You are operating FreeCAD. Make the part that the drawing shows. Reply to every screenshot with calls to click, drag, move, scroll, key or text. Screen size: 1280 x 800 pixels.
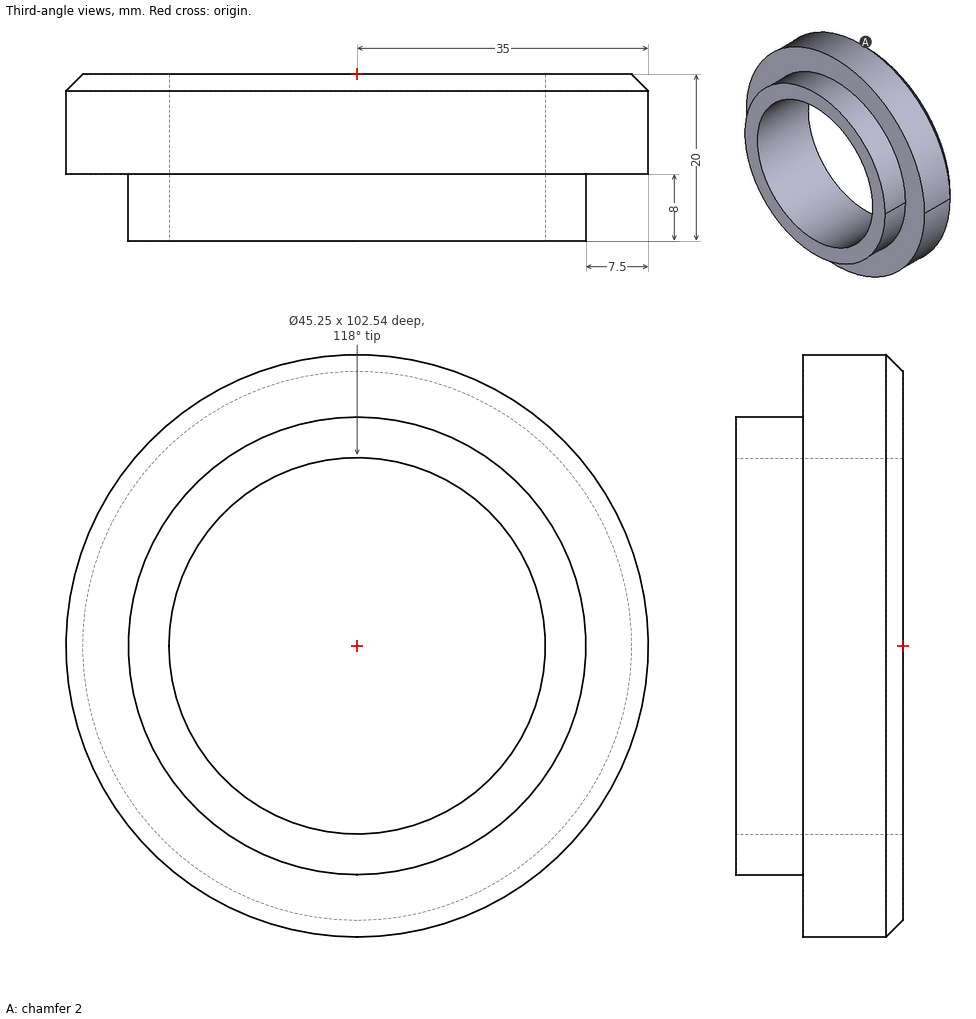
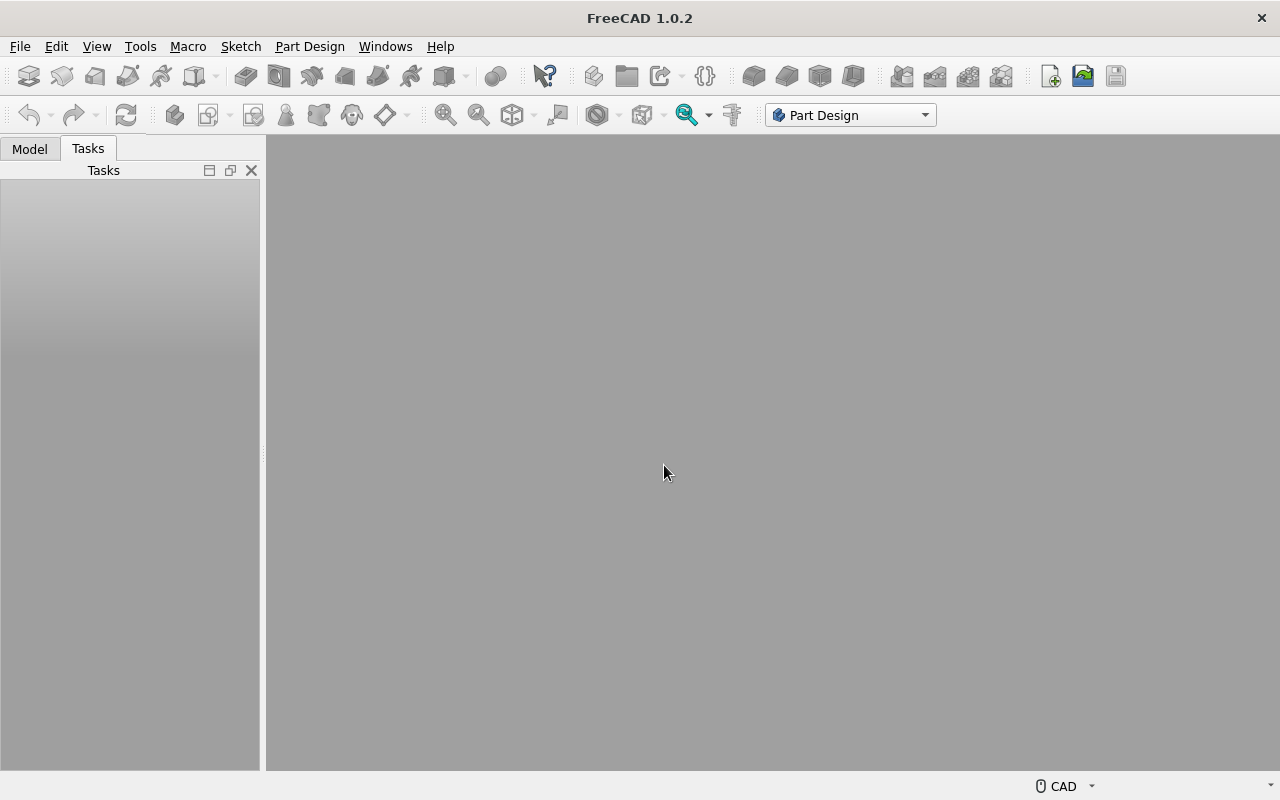
click(1050, 76)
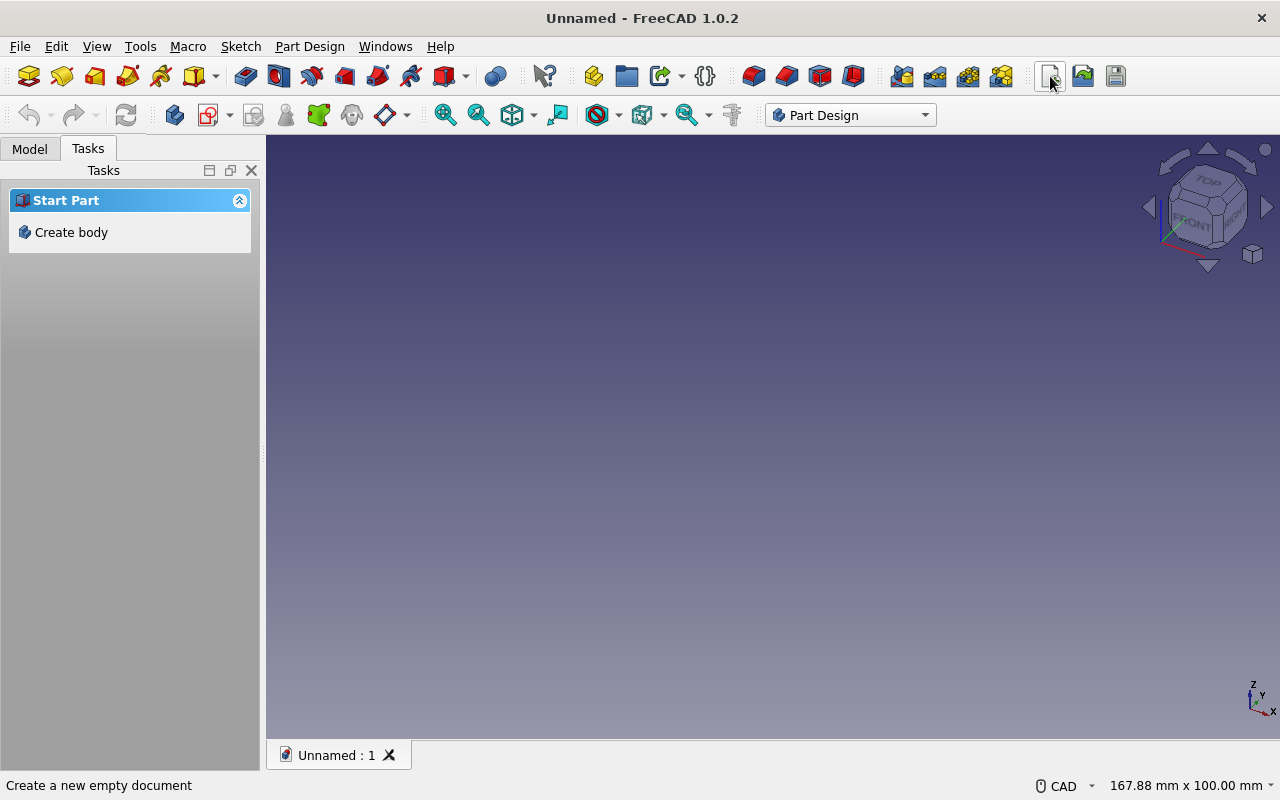
click(208, 116)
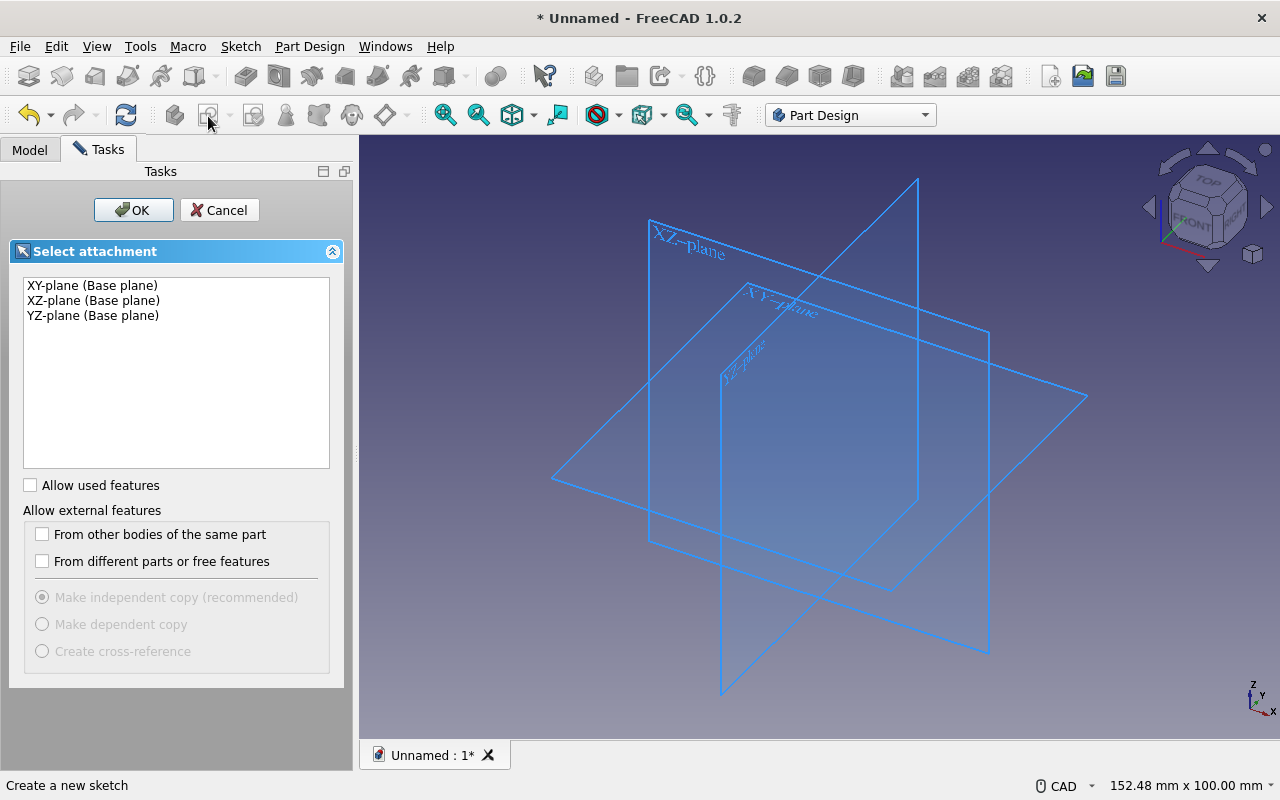
click(84, 286)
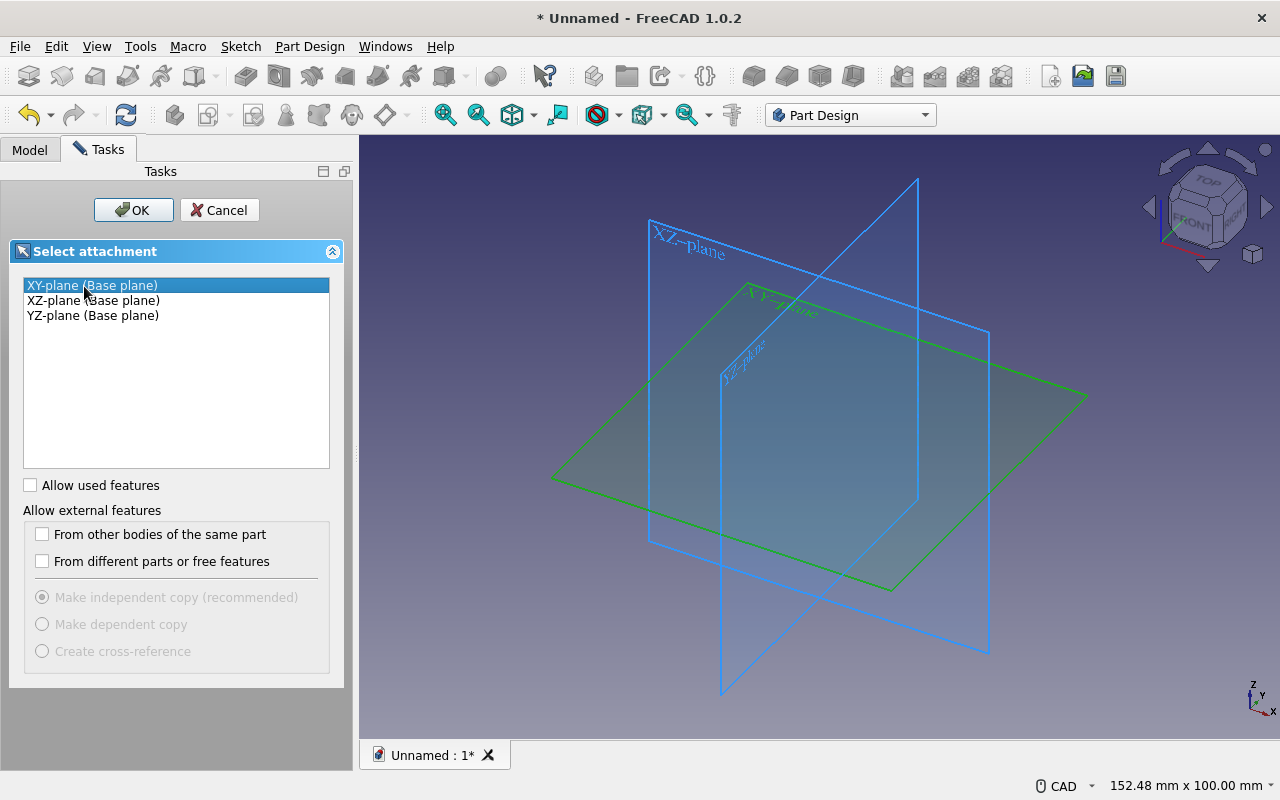
click(134, 210)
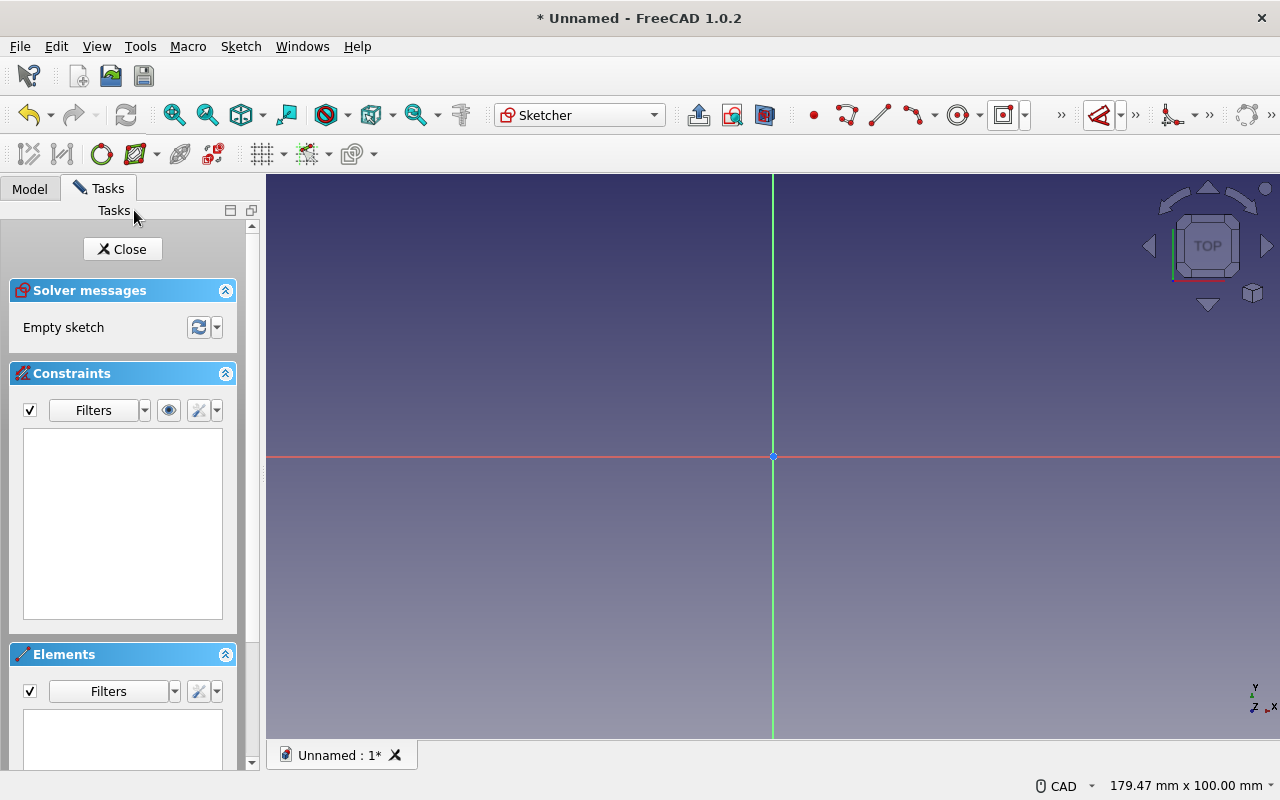
scroll(969, 546, up, 5)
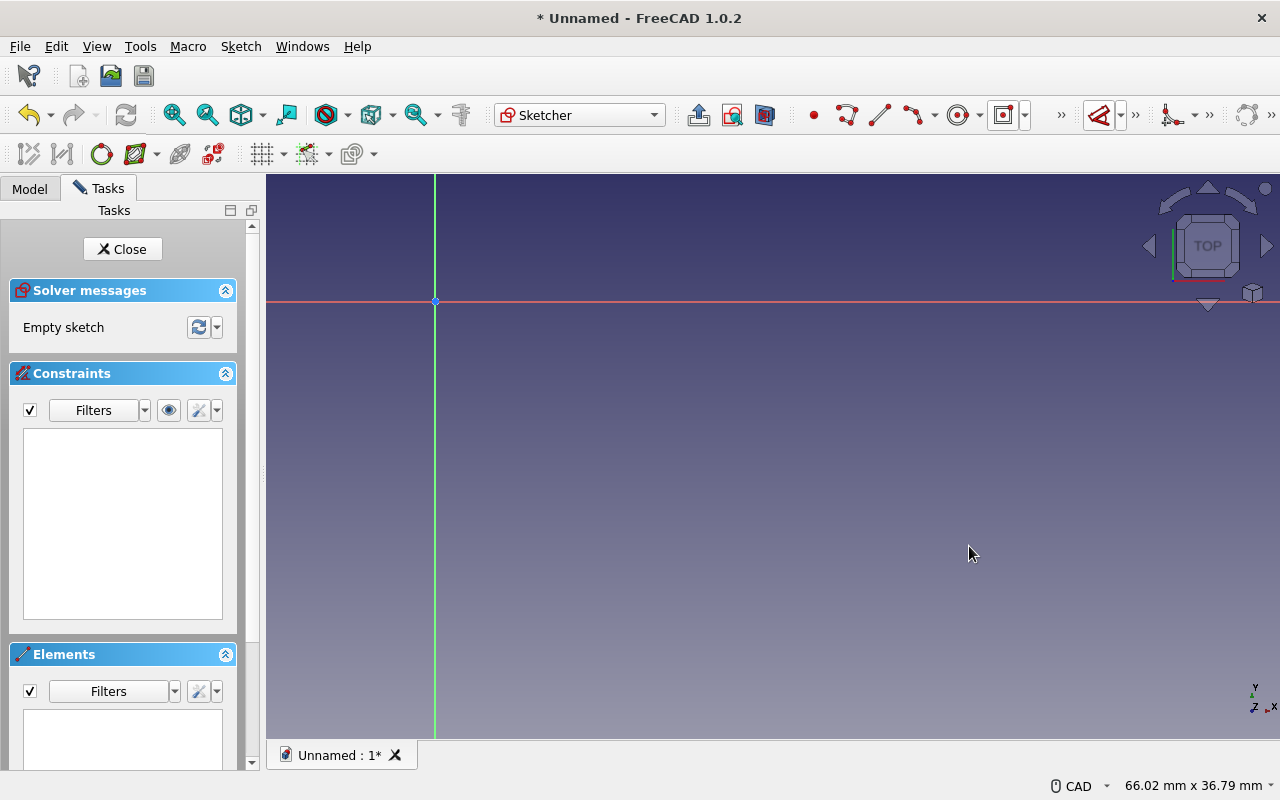
click(847, 116)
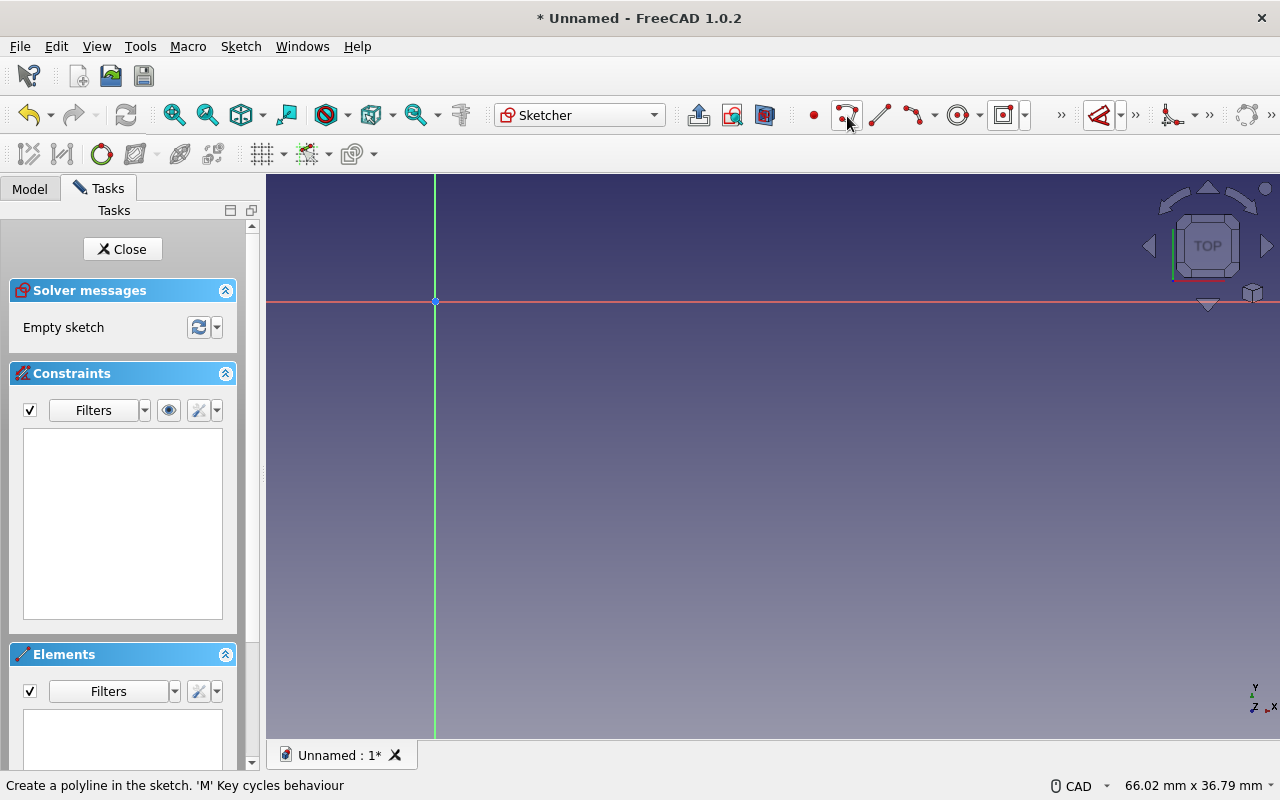
click(435, 302)
click(444, 609)
click(857, 609)
click(857, 486)
click(973, 486)
click(973, 311)
click(435, 302)
key(Escape)
key(Escape)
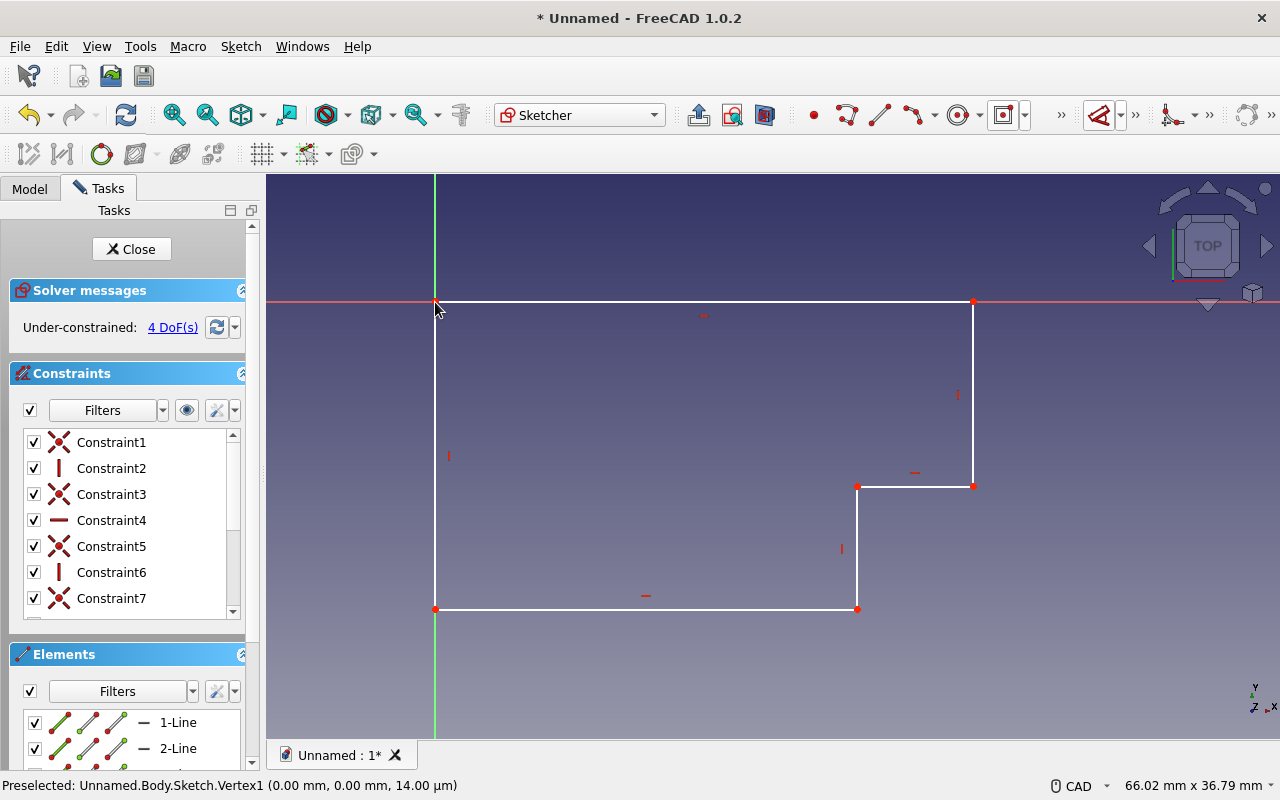
click(857, 573)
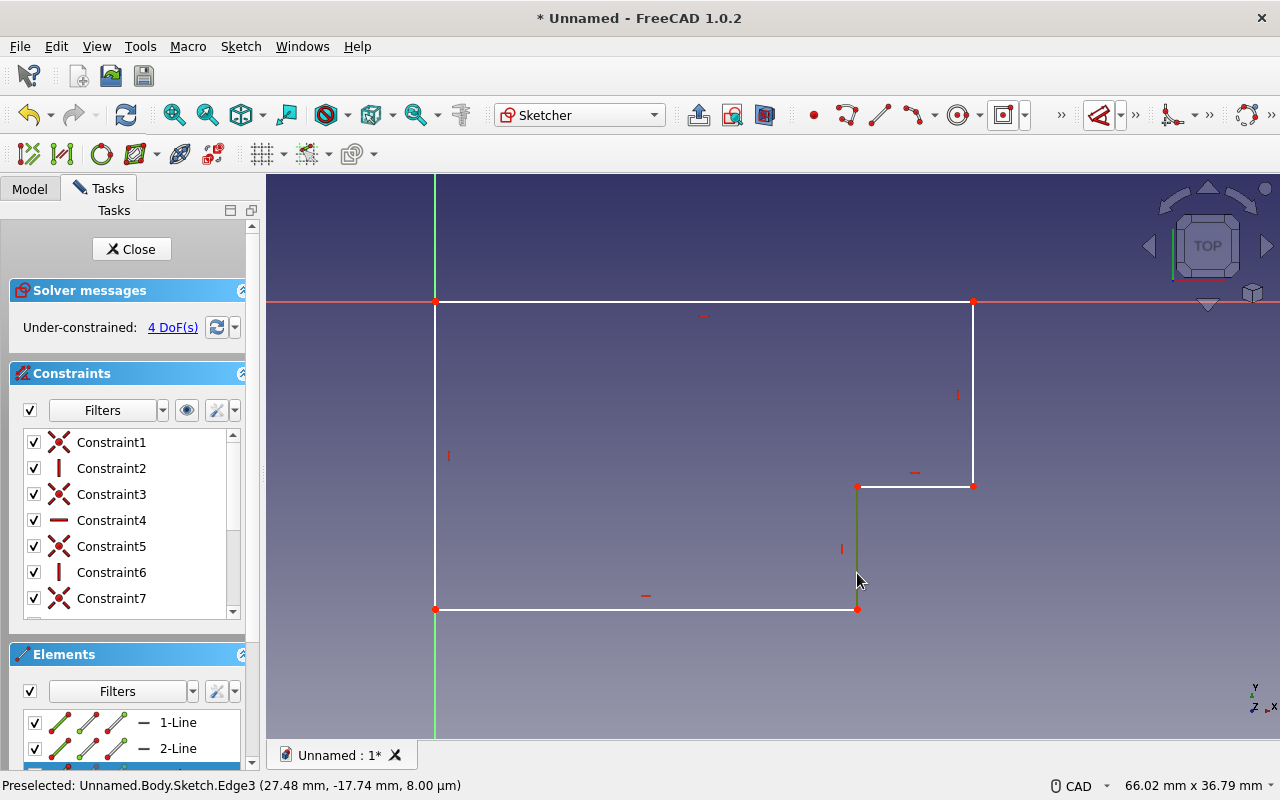
click(1120, 116)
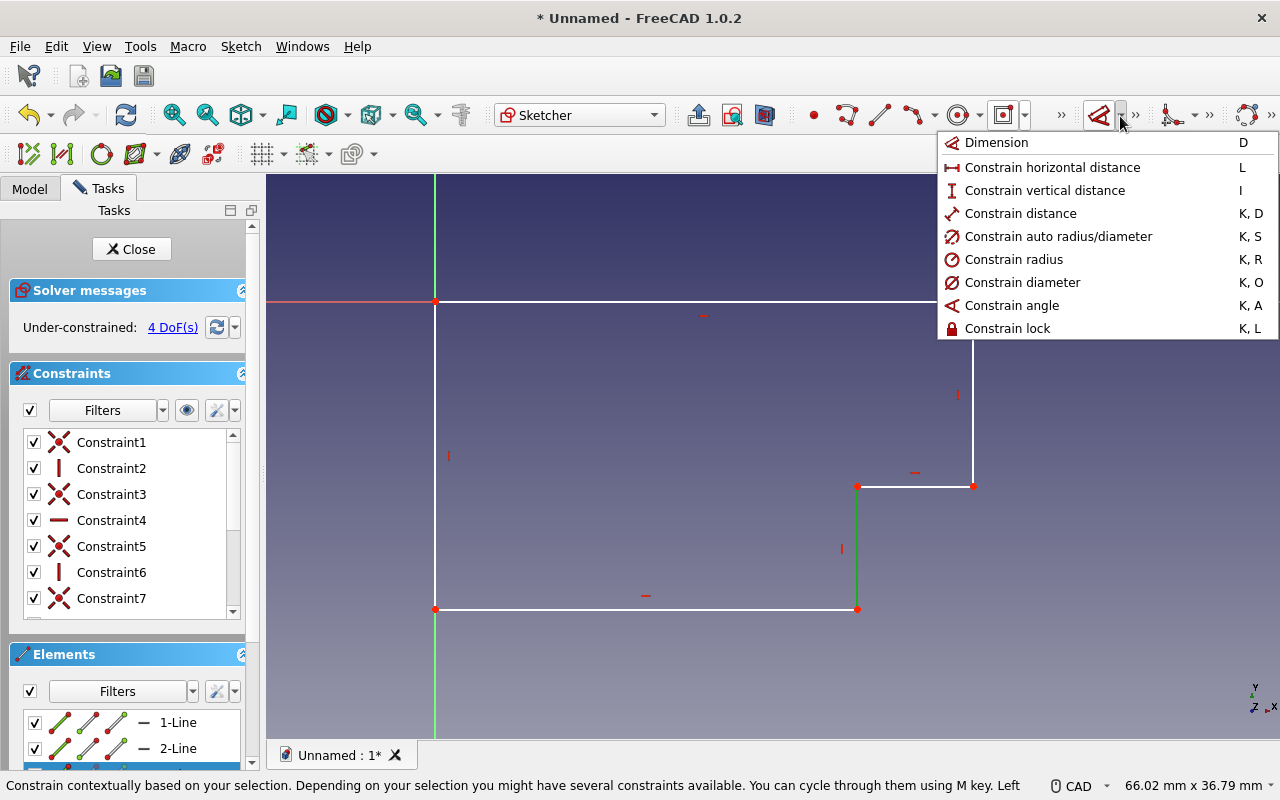
click(1108, 190)